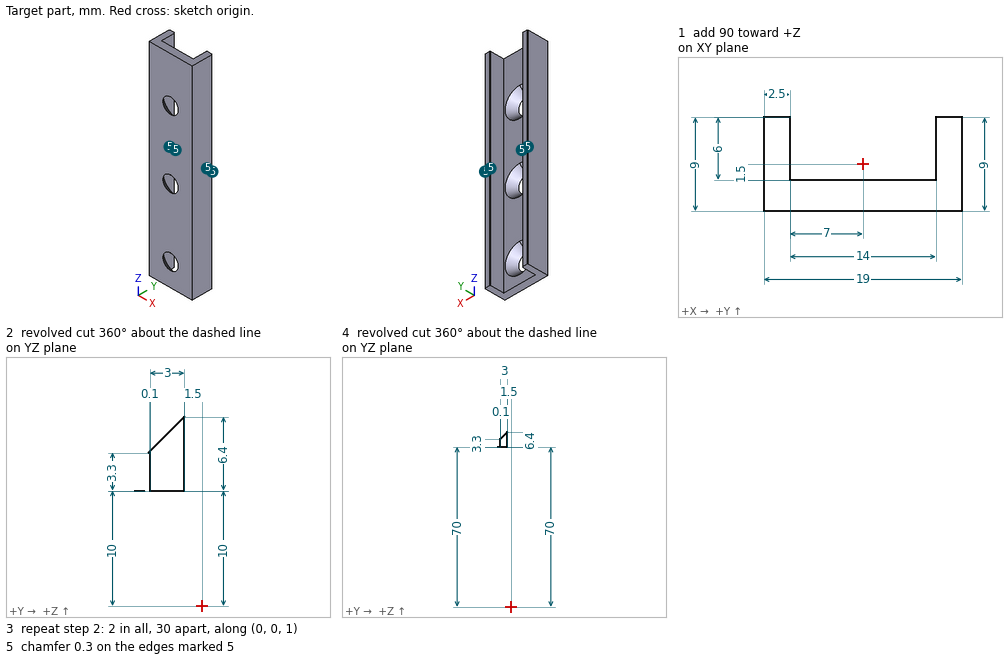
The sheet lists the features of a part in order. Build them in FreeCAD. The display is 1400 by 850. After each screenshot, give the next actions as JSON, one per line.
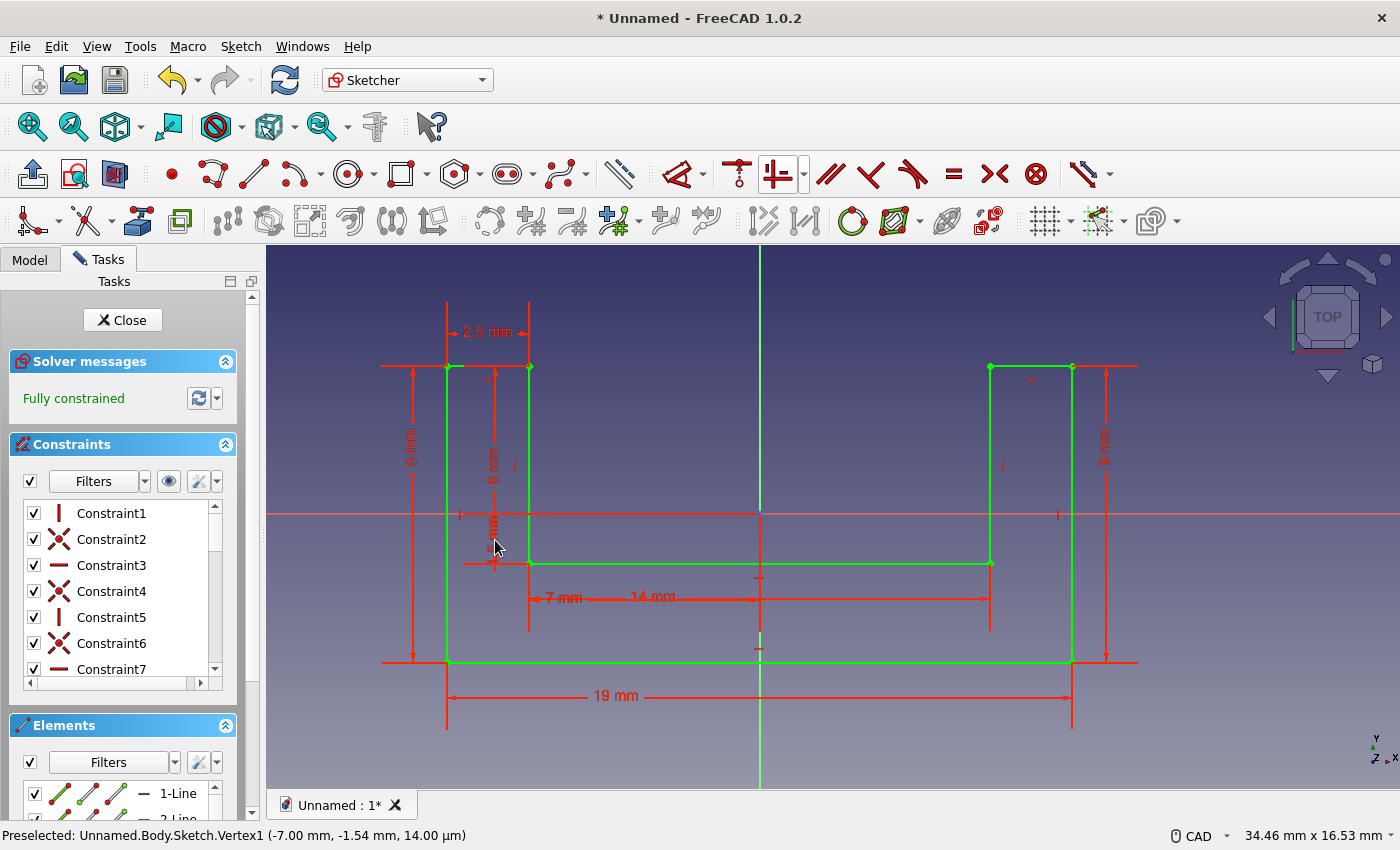
{"action": "left_click", "coordinate": [123, 320]}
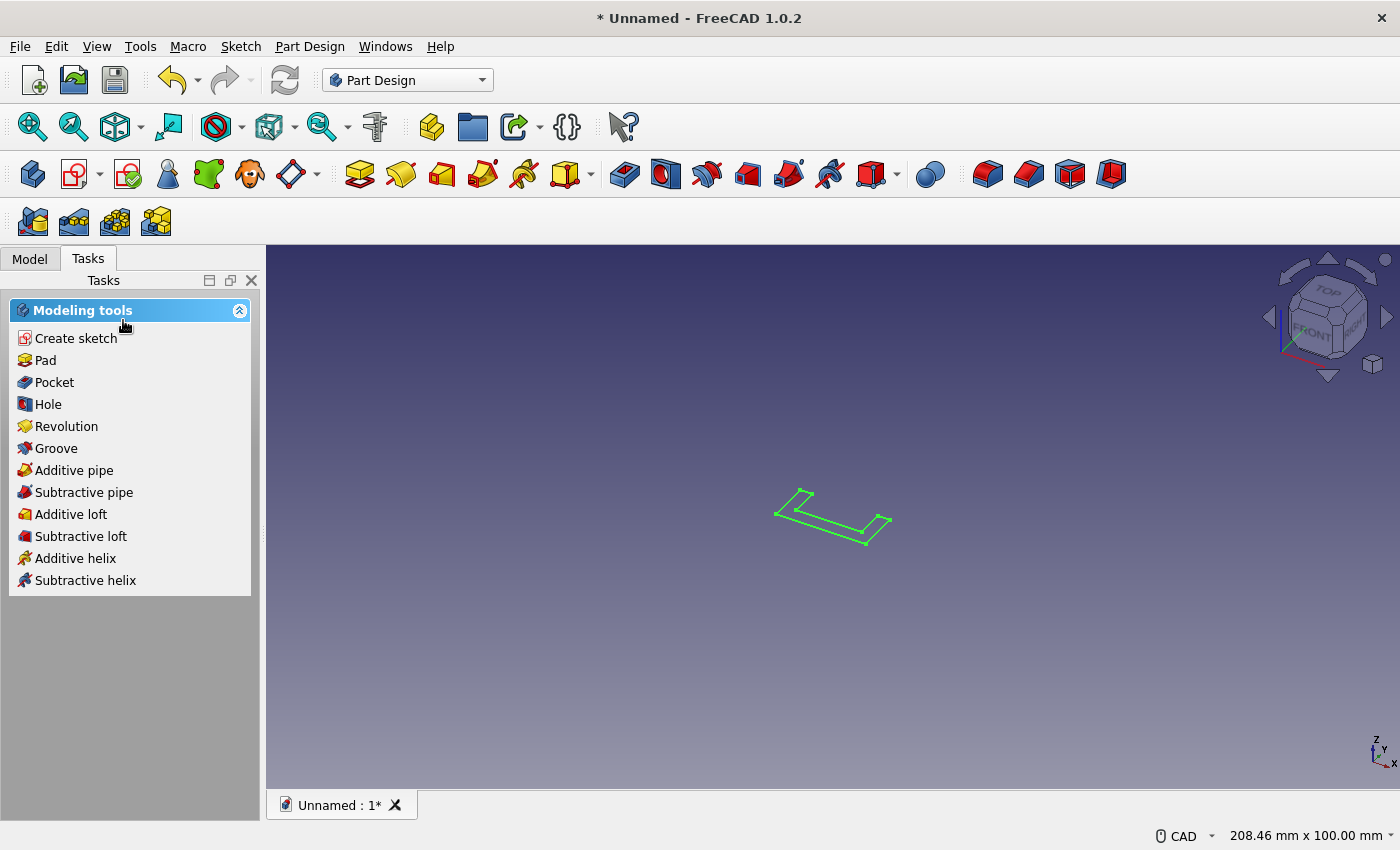
{"action": "left_click", "coordinate": [360, 174]}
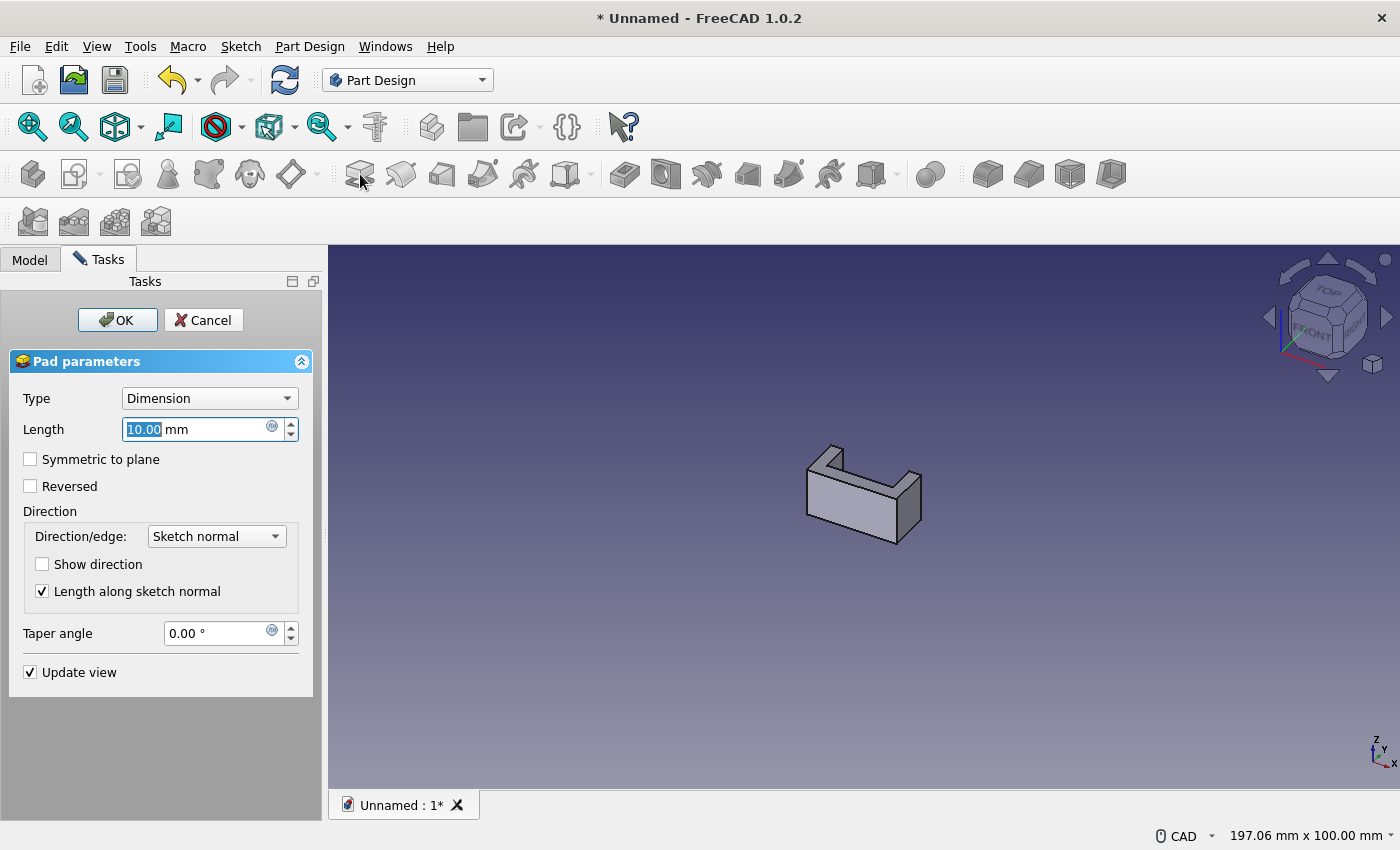
{"action": "type", "text": "90"}
{"action": "key", "text": "Tab"}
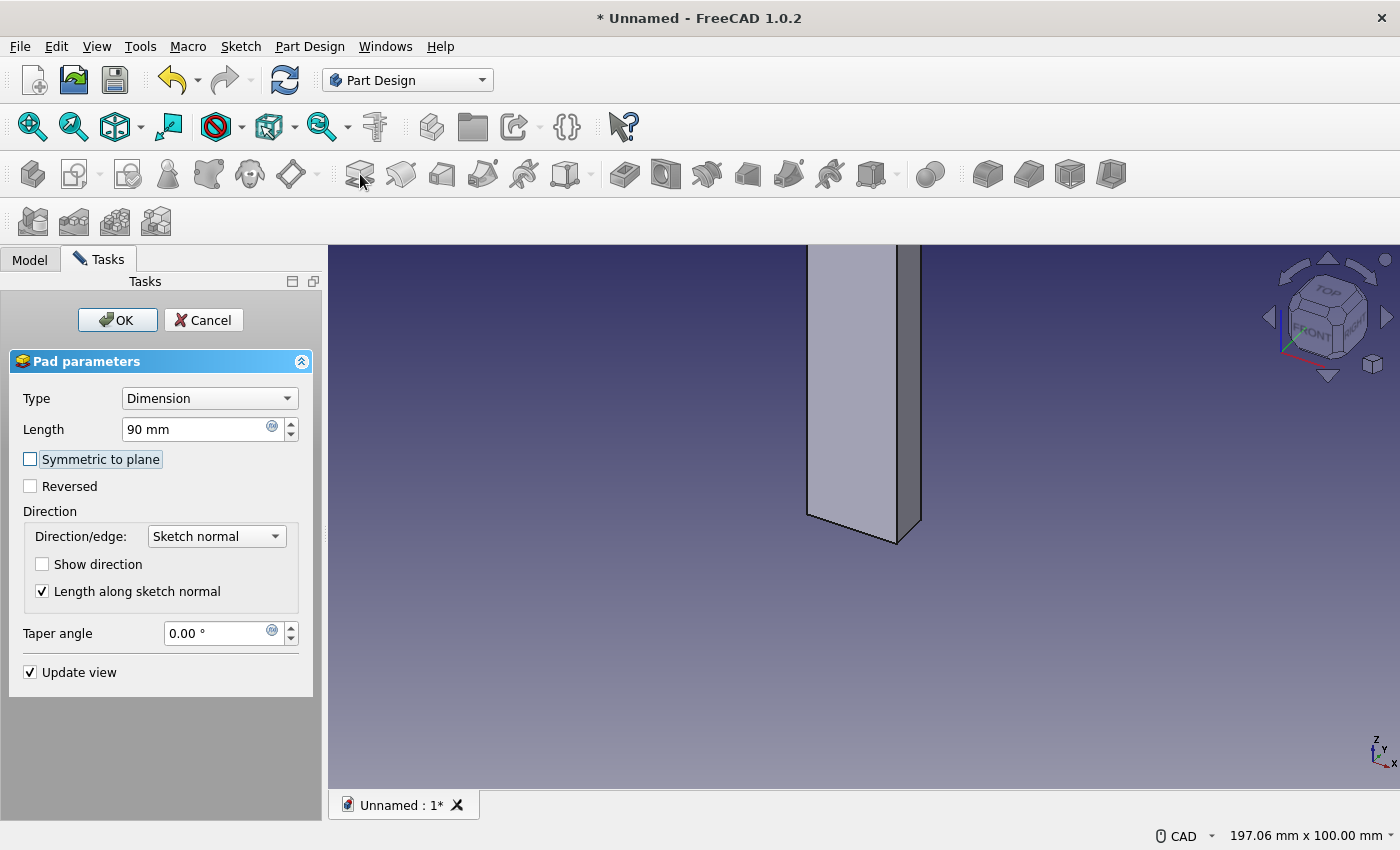
{"action": "left_click", "coordinate": [118, 320]}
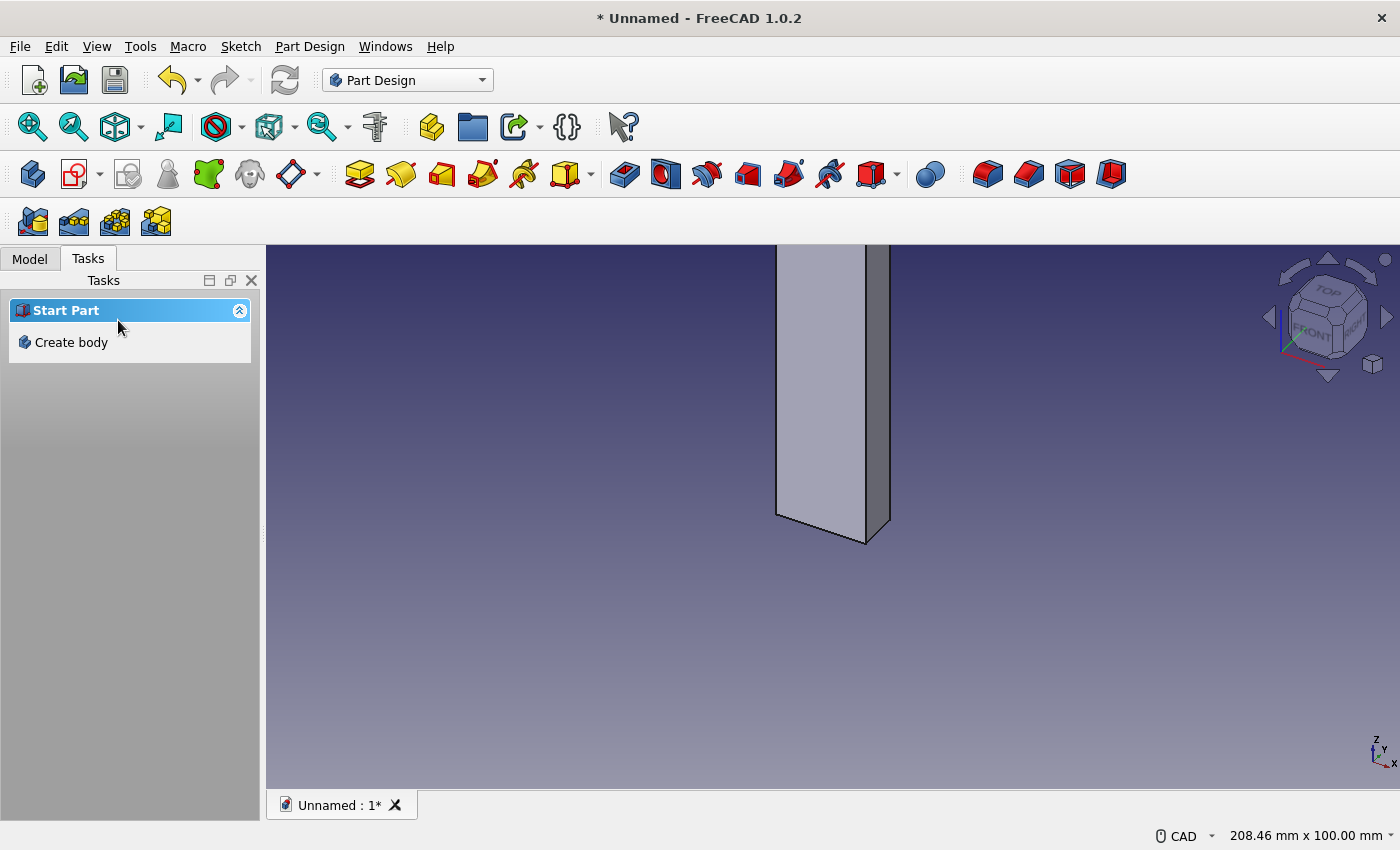
{"action": "left_click", "coordinate": [33, 128]}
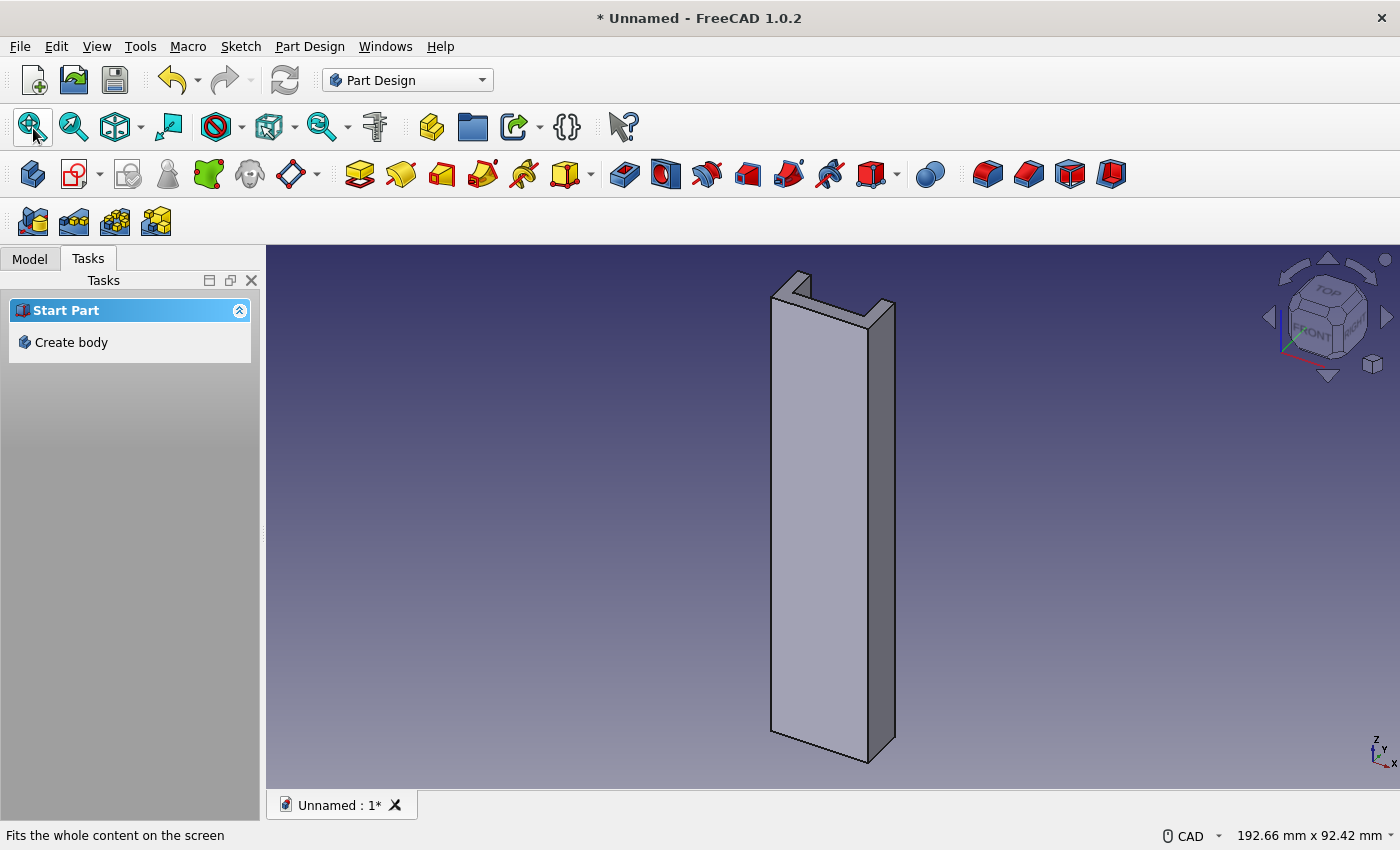
{"action": "left_click", "coordinate": [74, 174]}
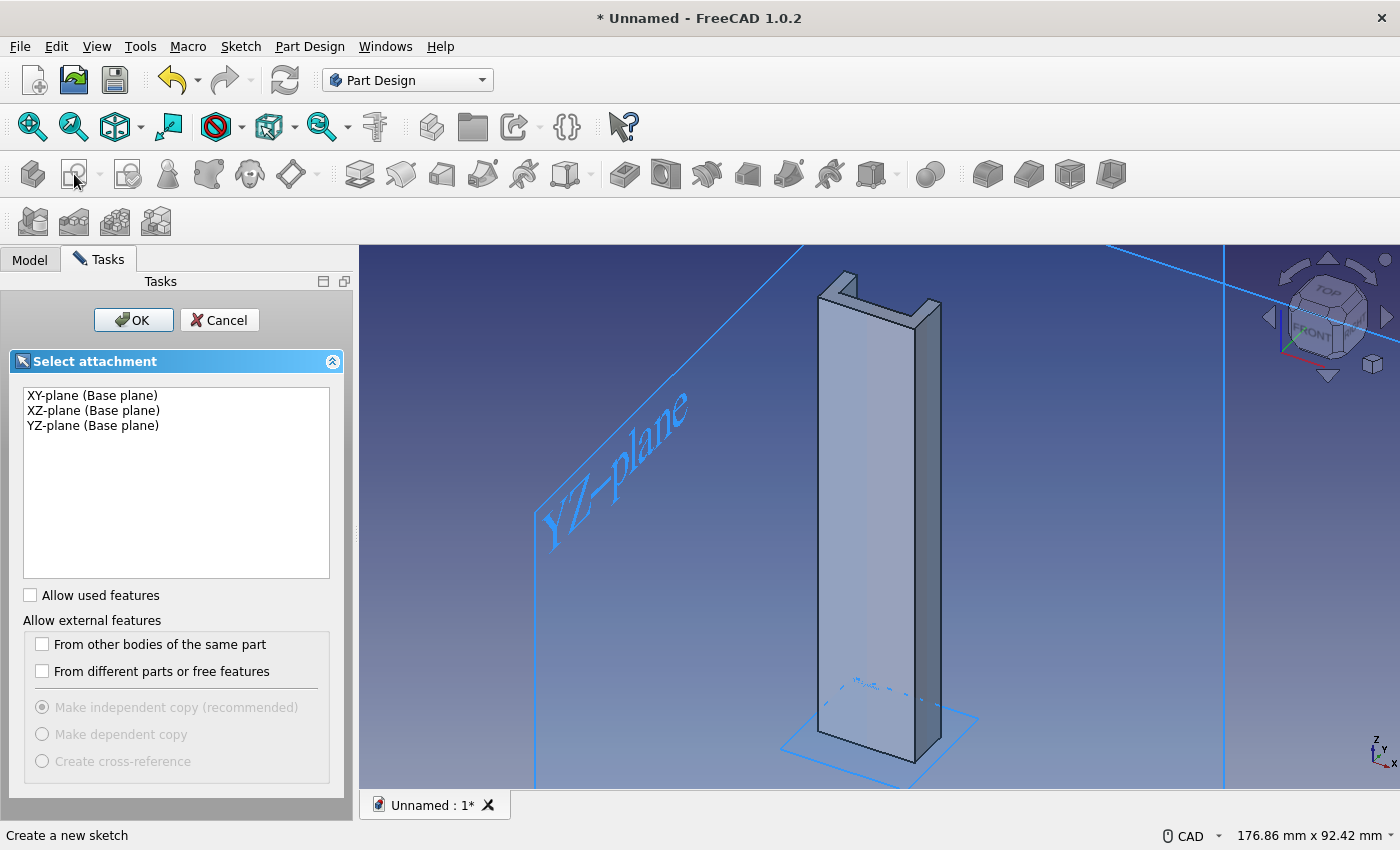
{"action": "left_click", "coordinate": [84, 426]}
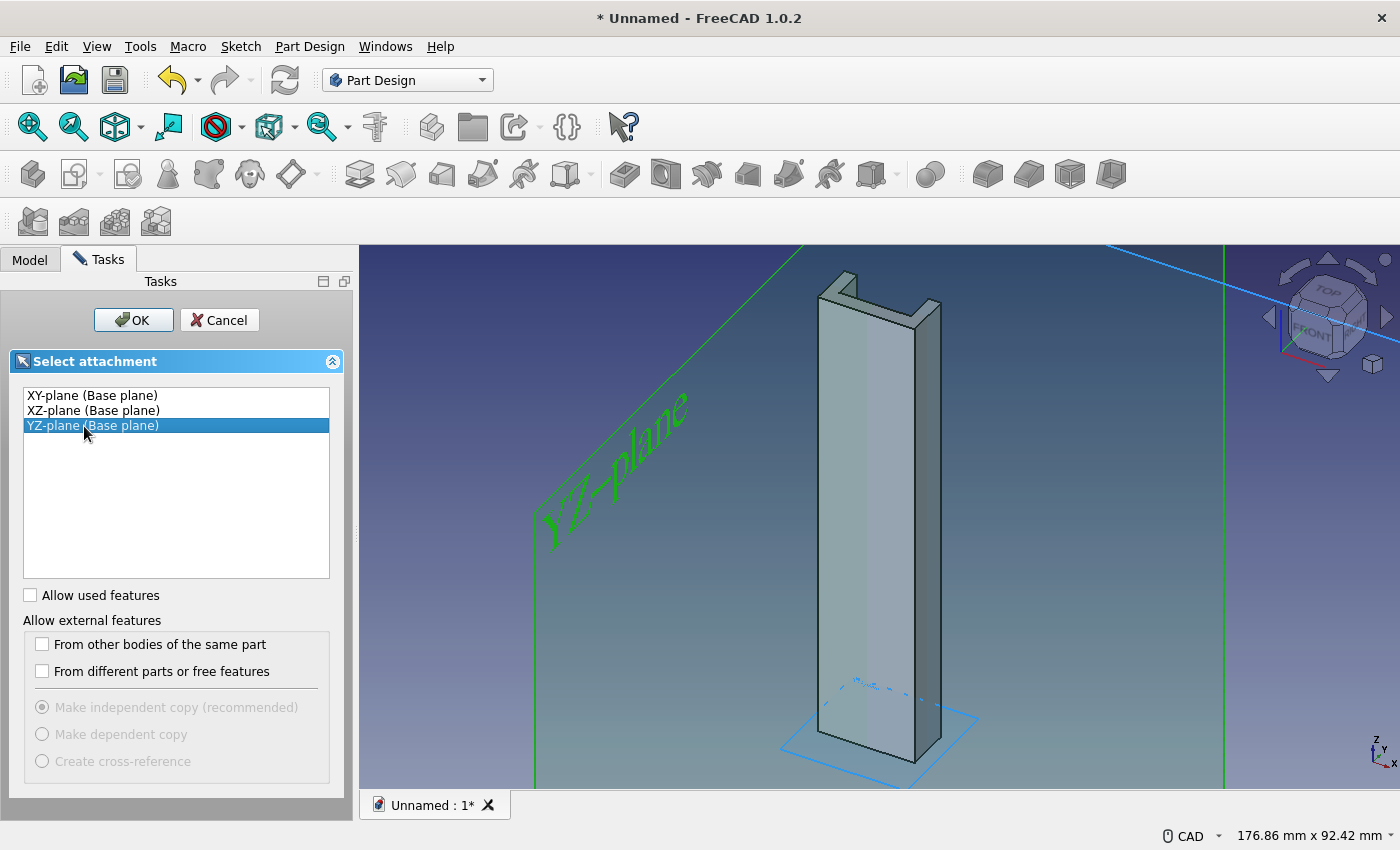
{"action": "left_click", "coordinate": [134, 320]}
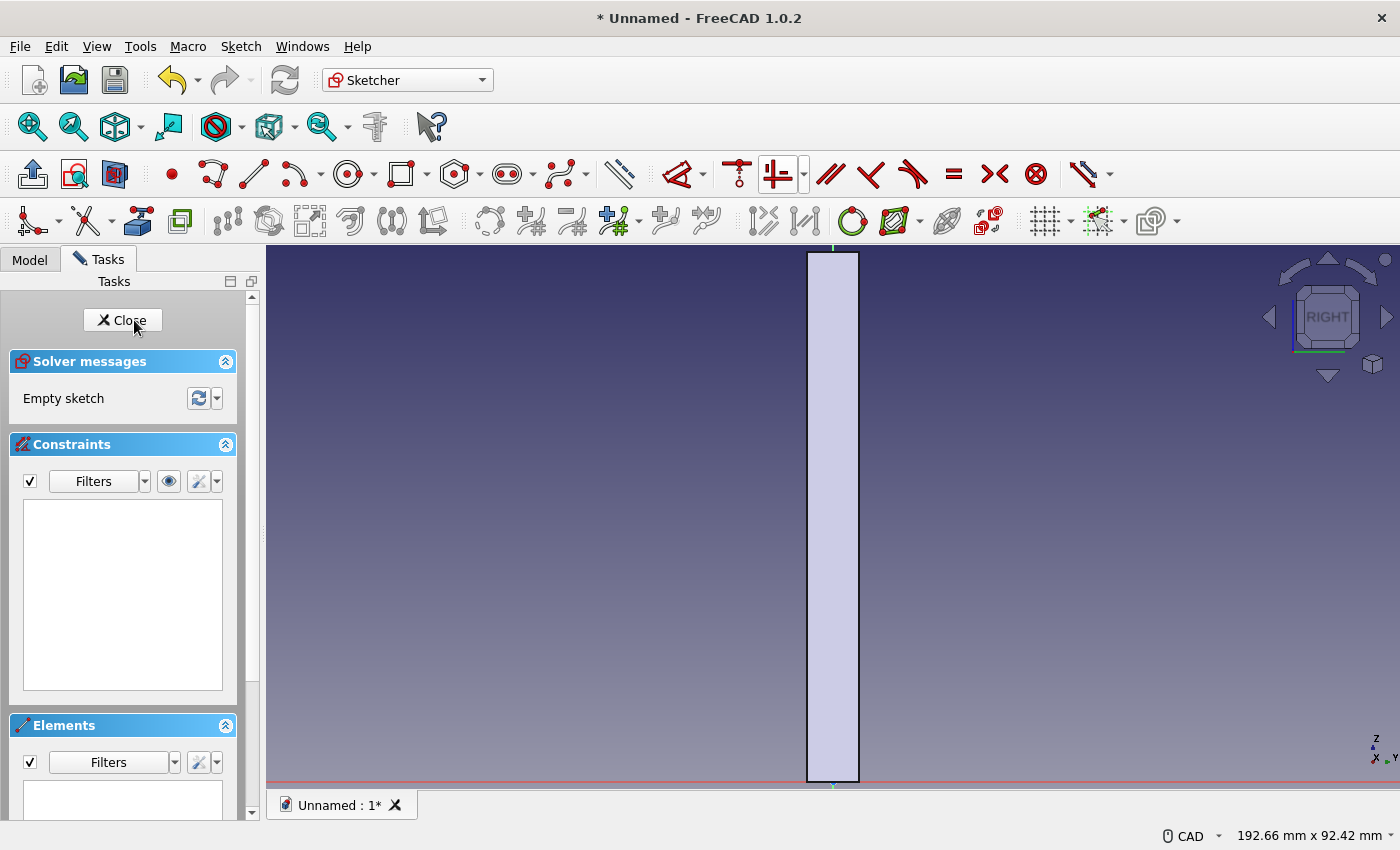
{"action": "left_click", "coordinate": [115, 174]}